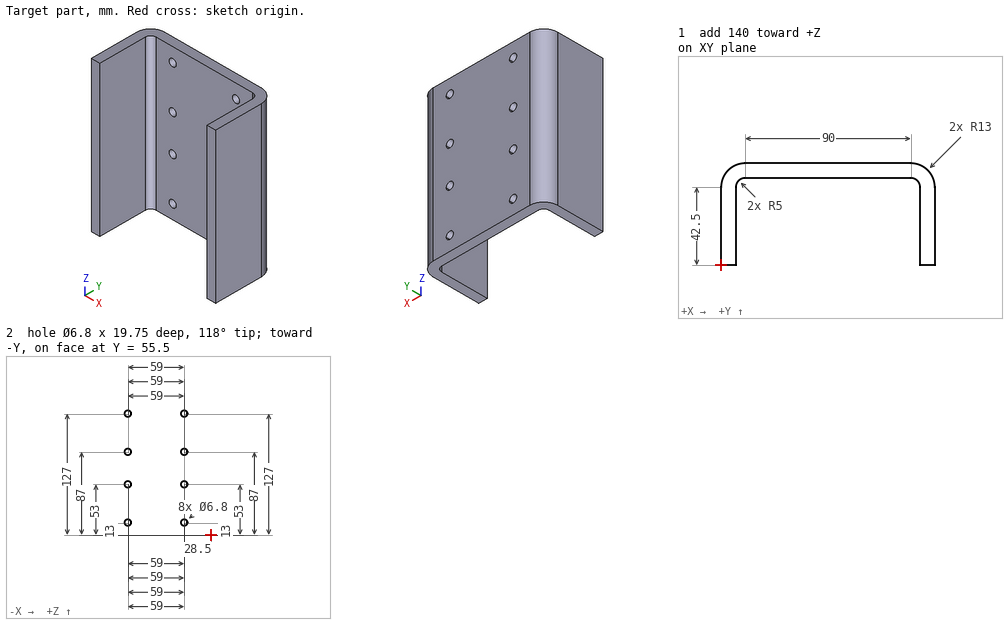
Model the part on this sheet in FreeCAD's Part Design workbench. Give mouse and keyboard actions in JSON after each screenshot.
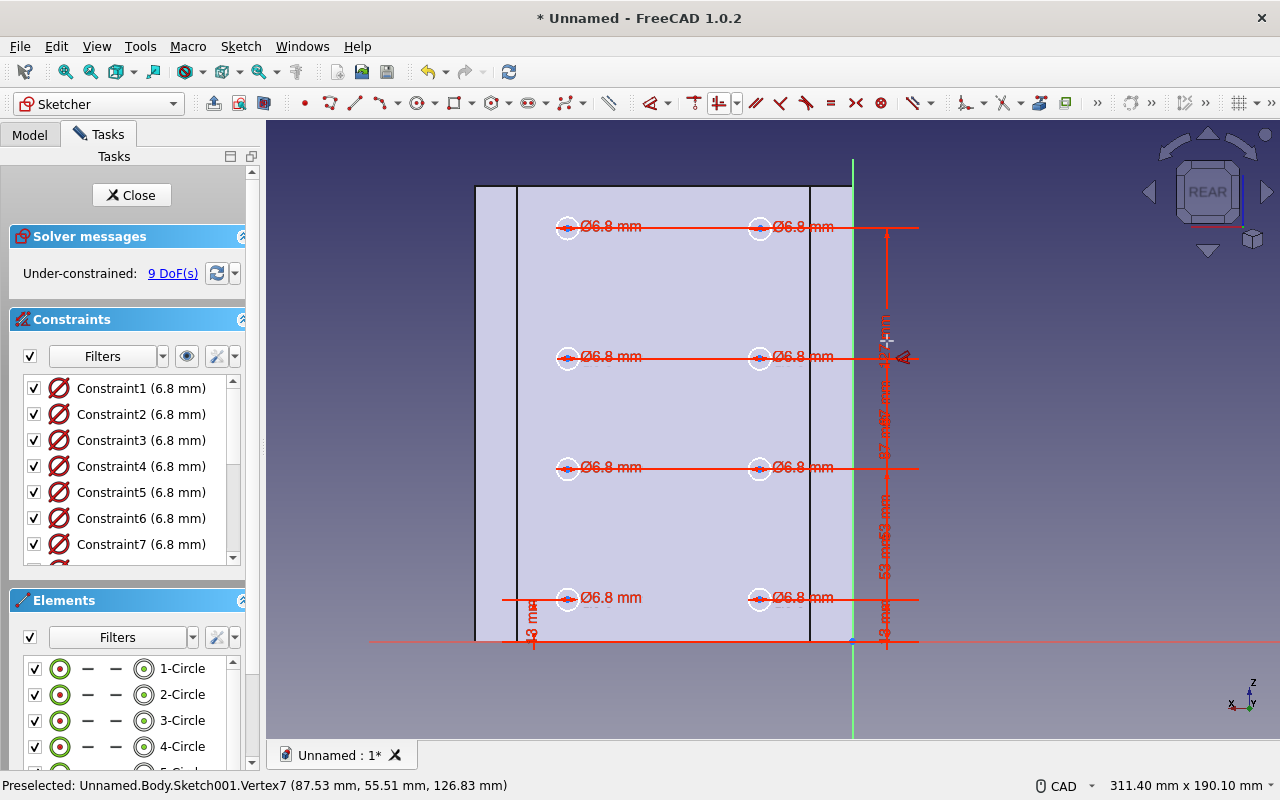
{"action": "left_click", "coordinate": [760, 229]}
{"action": "left_click", "coordinate": [887, 291]}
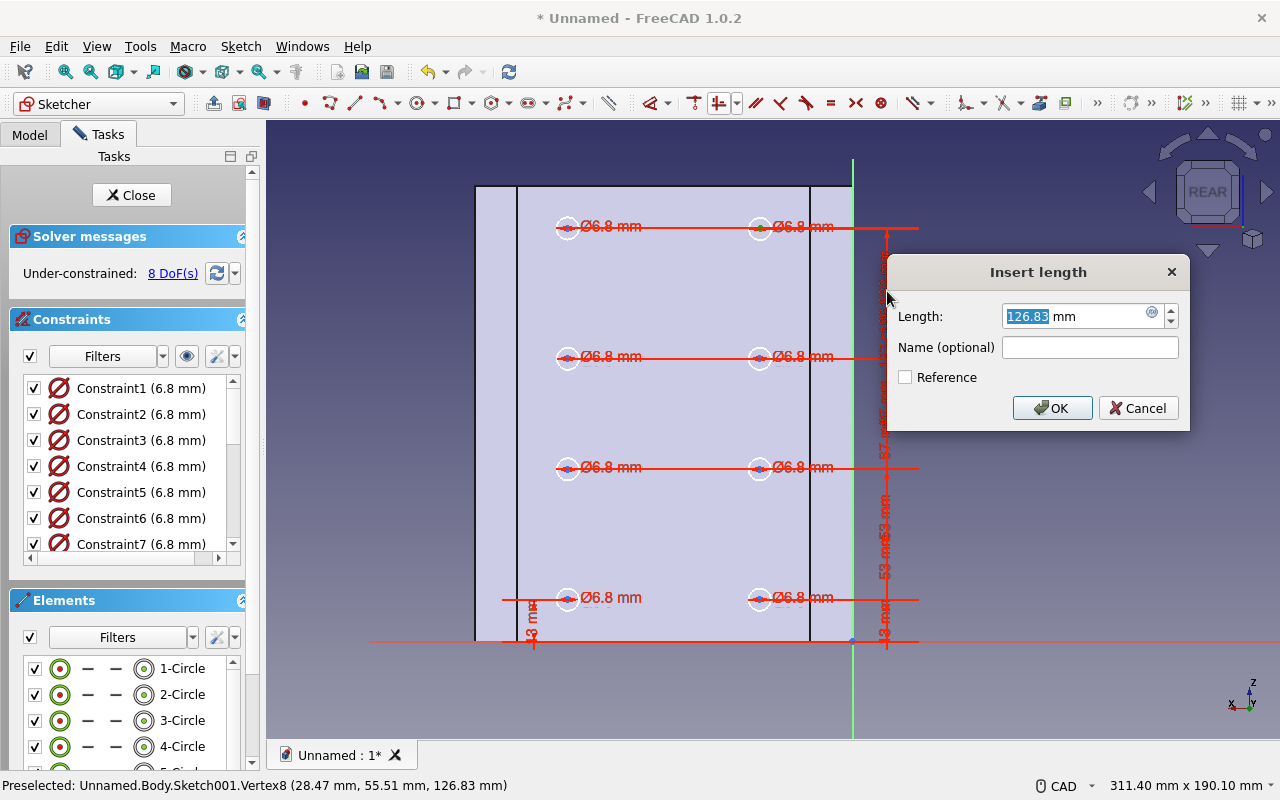
{"action": "type", "text": "127"}
{"action": "key", "text": "Return"}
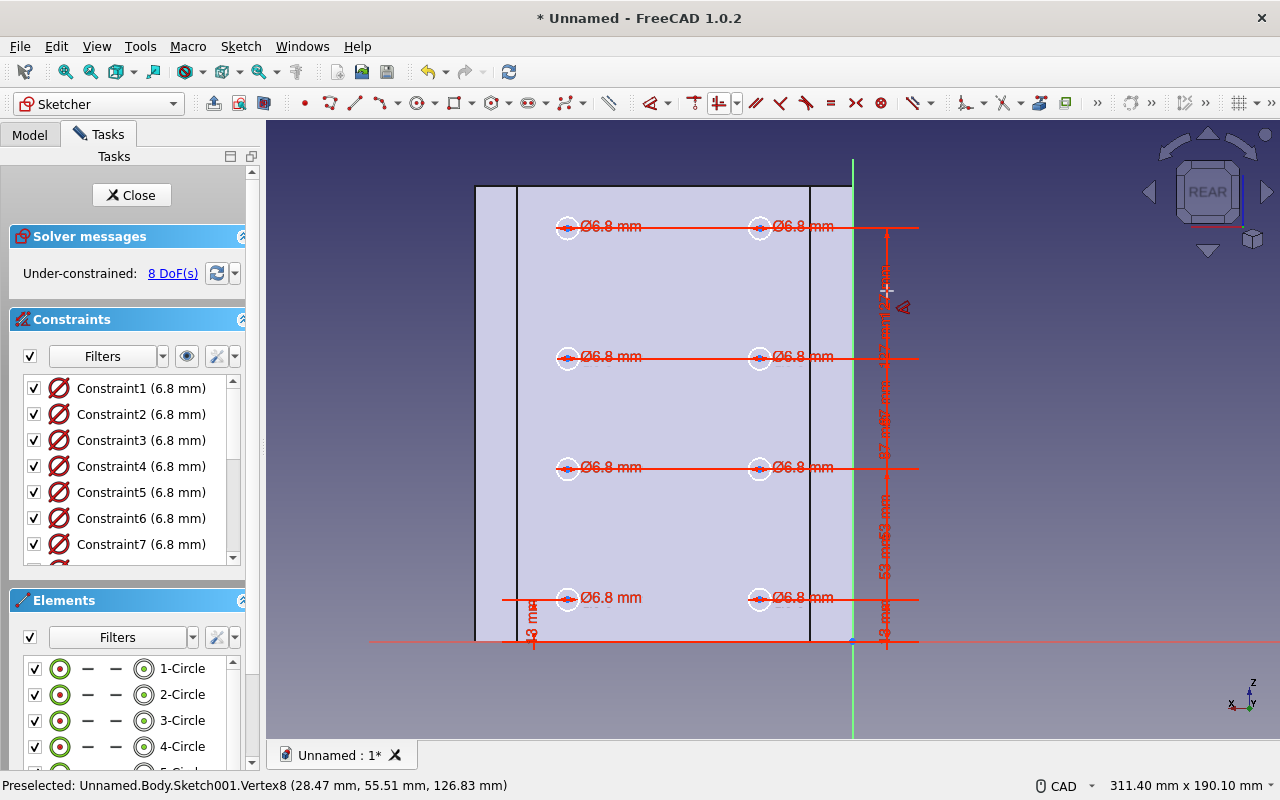
{"action": "left_click", "coordinate": [760, 600]}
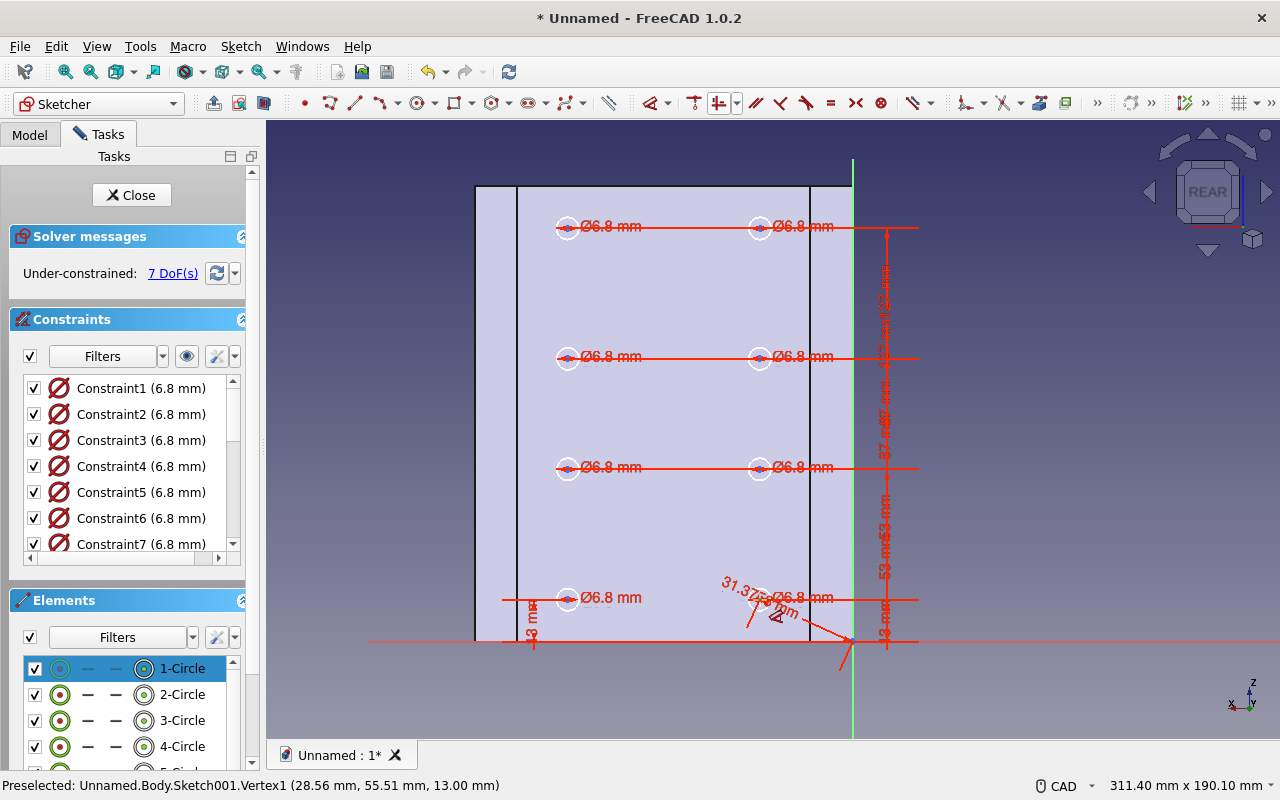
{"action": "left_click", "coordinate": [568, 600]}
{"action": "left_click", "coordinate": [664, 566]}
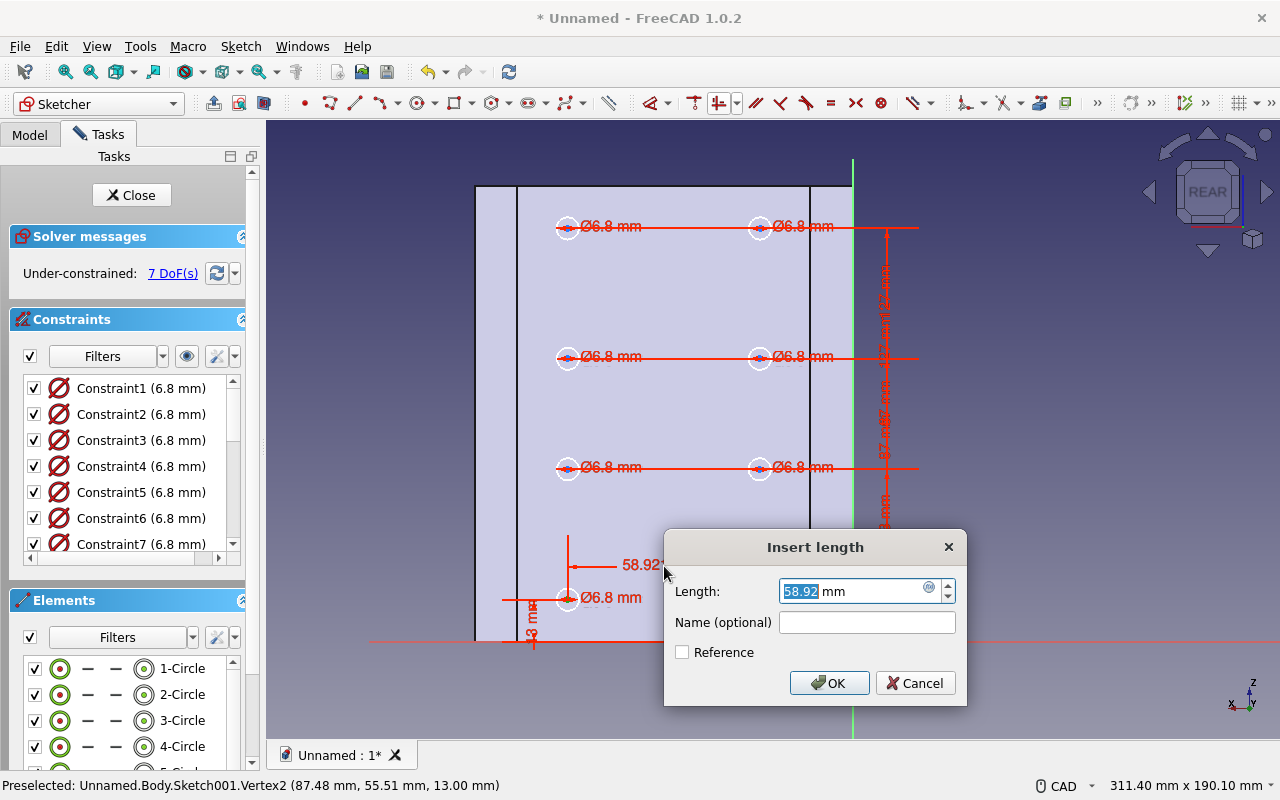
{"action": "type", "text": "59"}
{"action": "key", "text": "Return"}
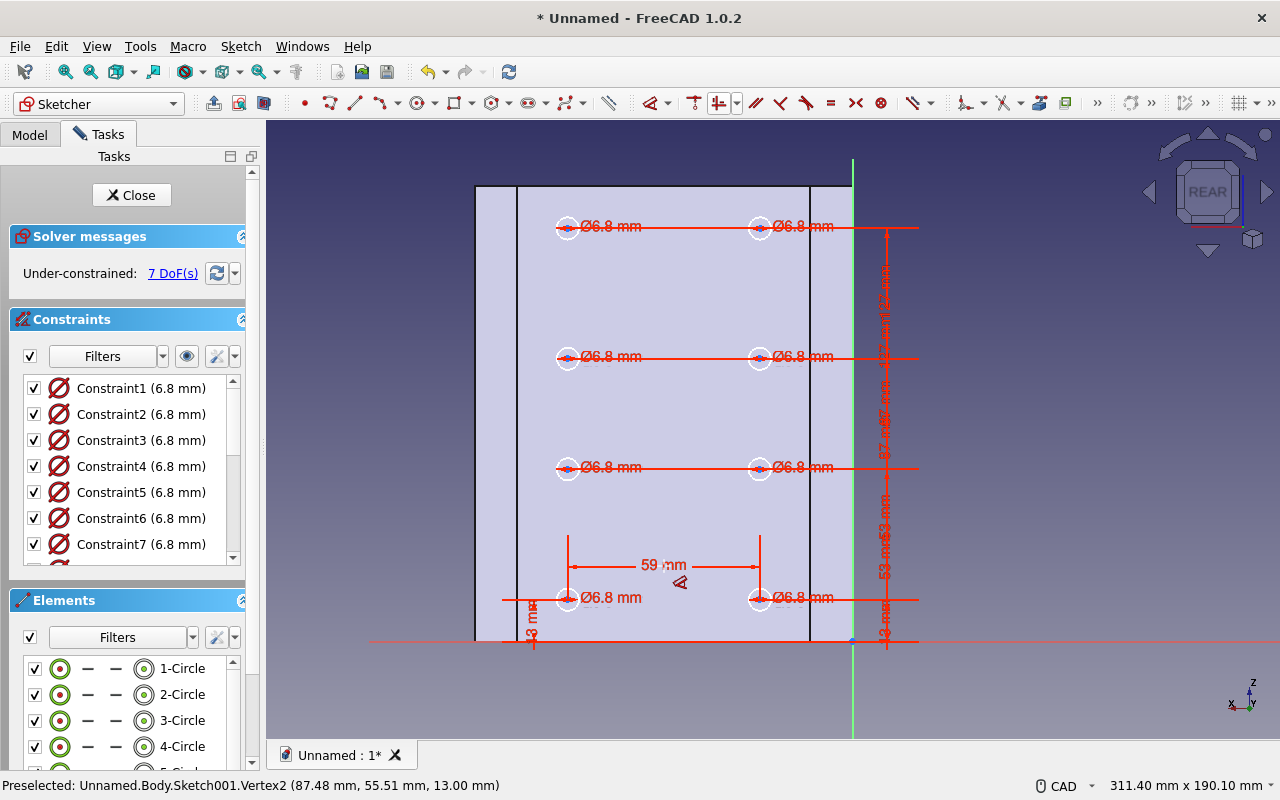
{"action": "left_click", "coordinate": [760, 600]}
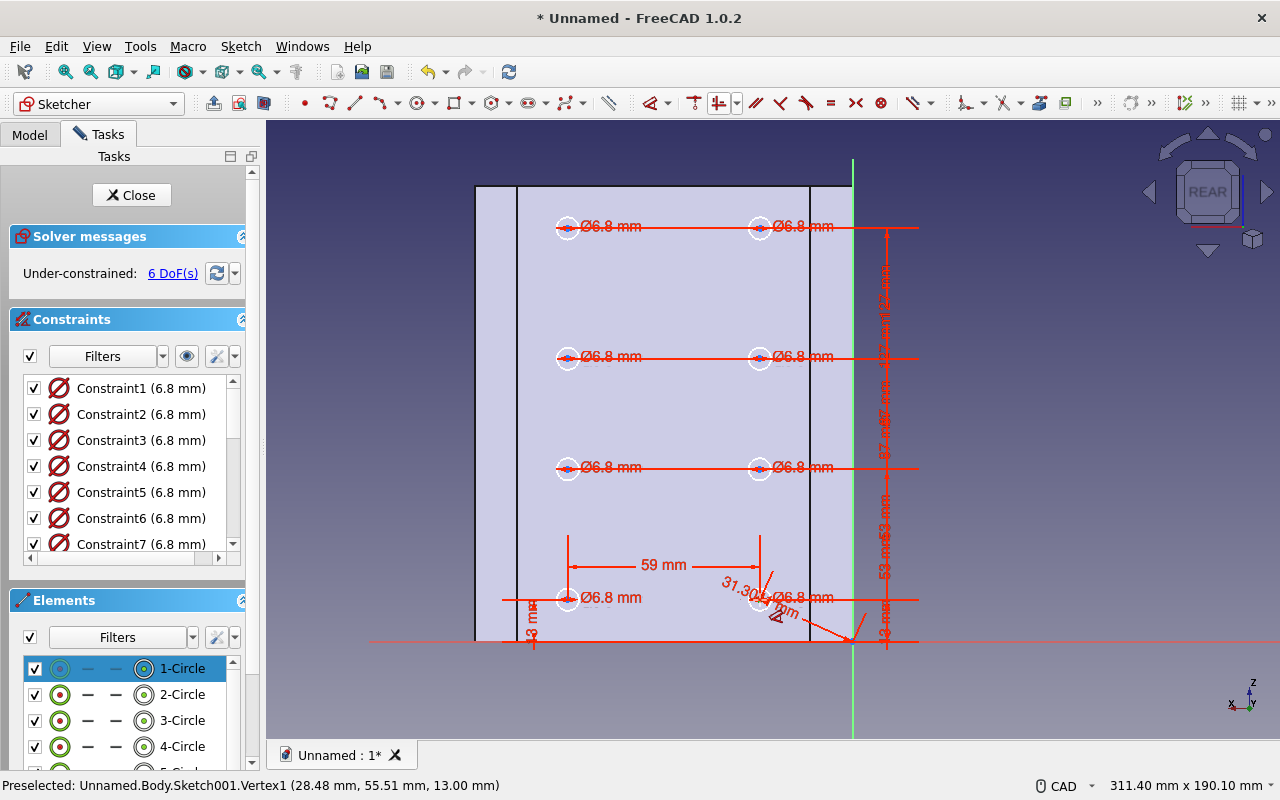
{"action": "left_click", "coordinate": [568, 469]}
{"action": "left_click", "coordinate": [664, 435]}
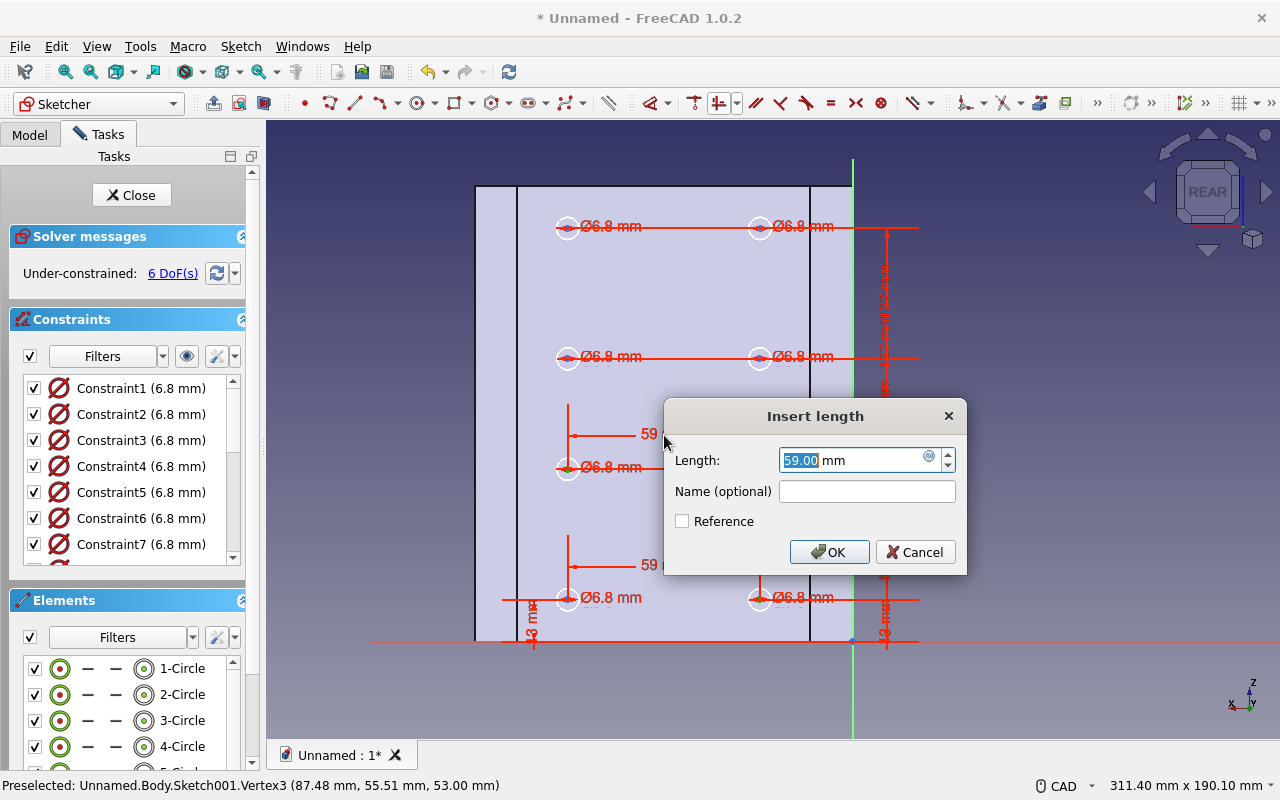
{"action": "type", "text": "59"}
{"action": "key", "text": "Return"}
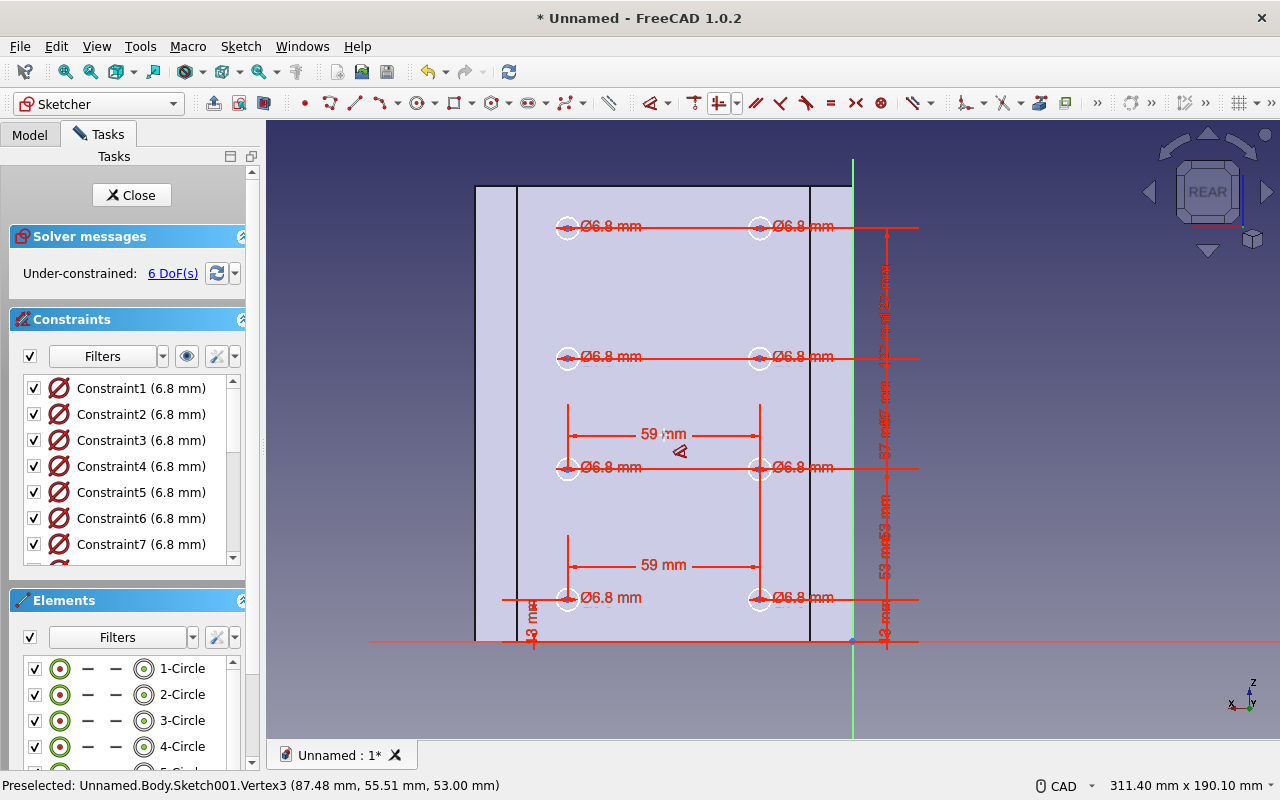
{"action": "left_click", "coordinate": [568, 469]}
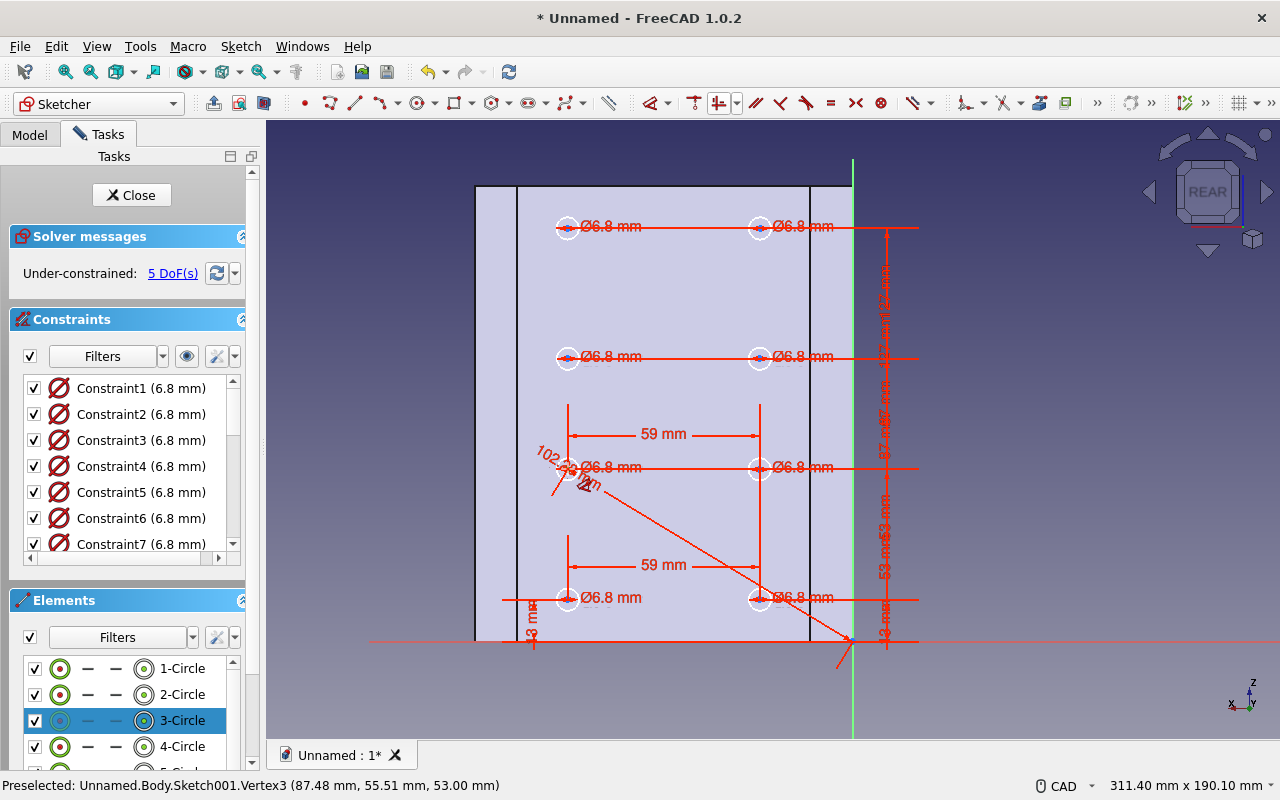
{"action": "left_click", "coordinate": [760, 469]}
{"action": "left_click", "coordinate": [664, 503]}